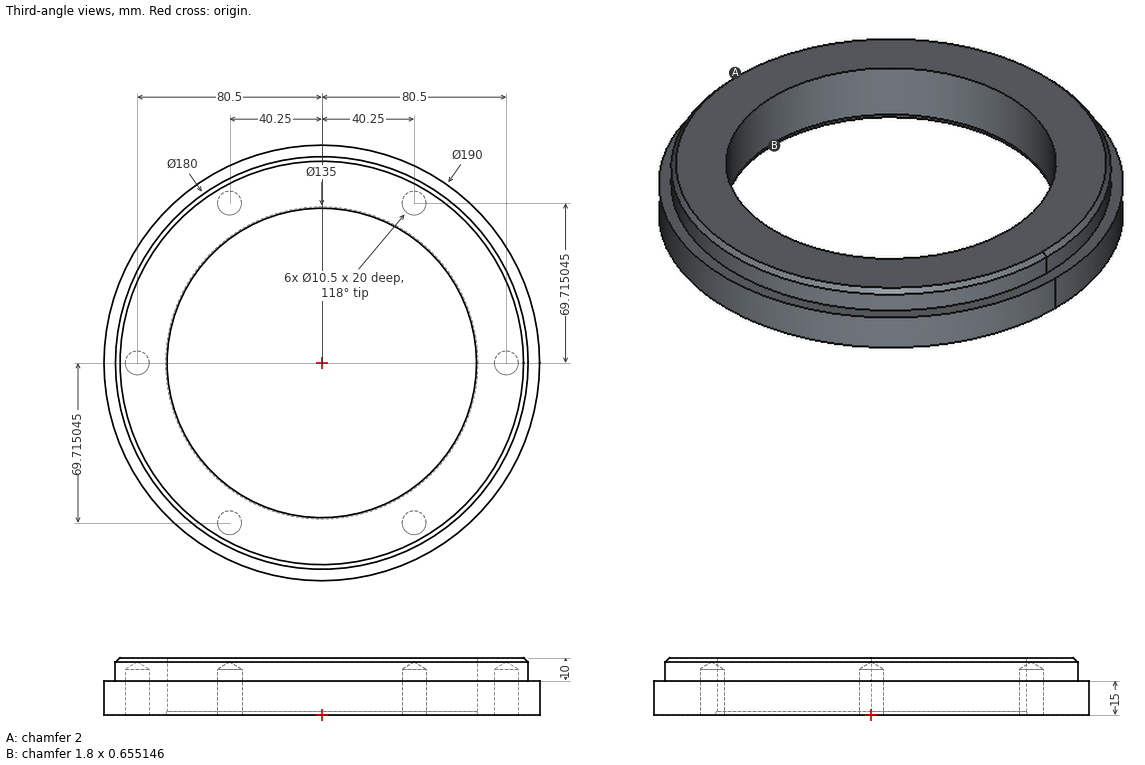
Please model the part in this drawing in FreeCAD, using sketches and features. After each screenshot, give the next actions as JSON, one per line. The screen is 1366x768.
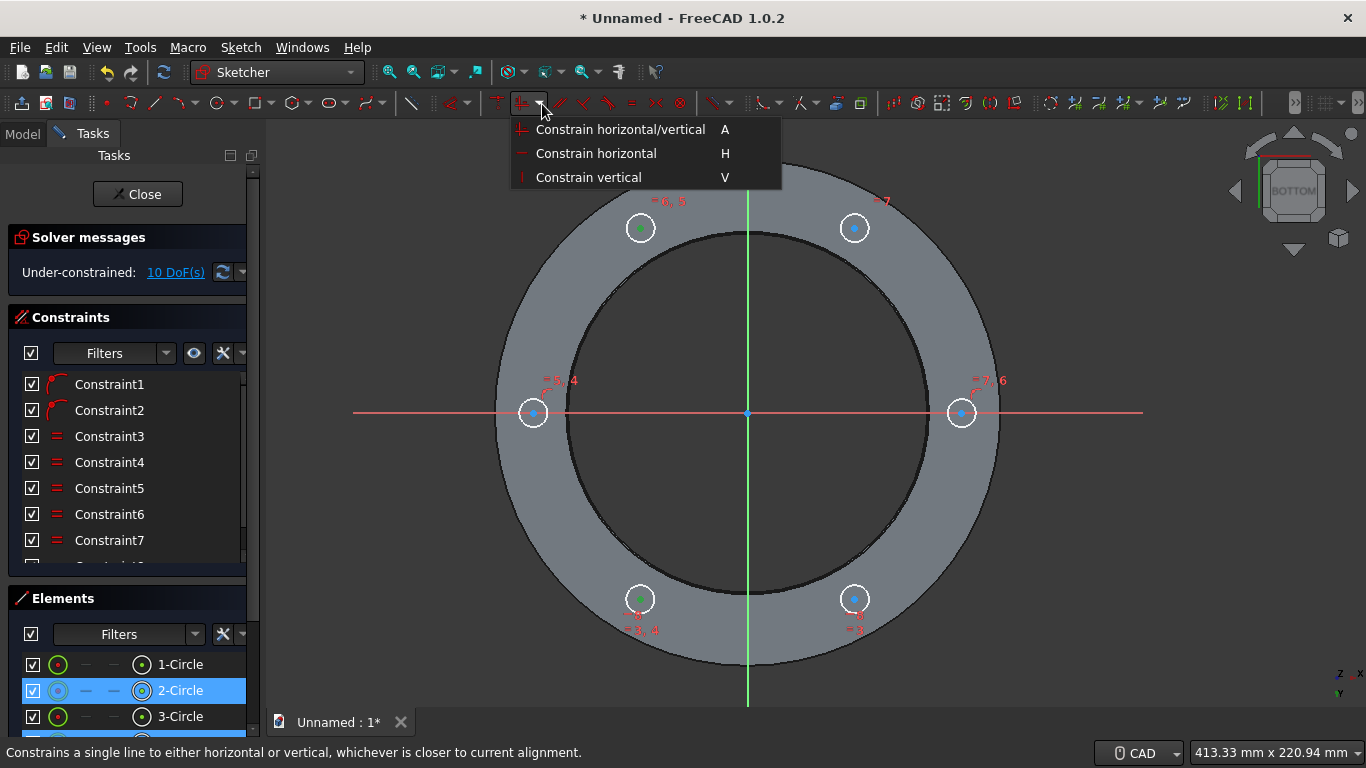
{"action": "left_click", "coordinate": [646, 177]}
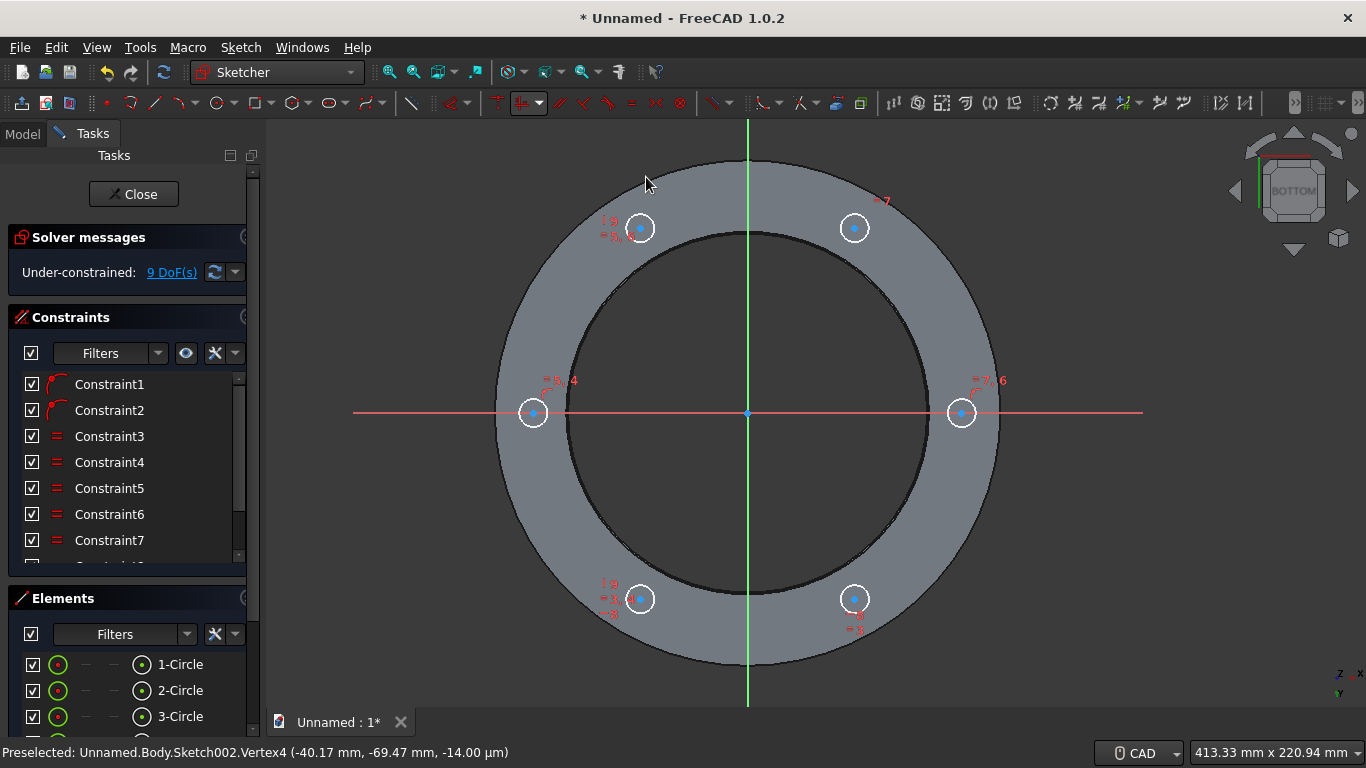
{"action": "left_click", "coordinate": [855, 599]}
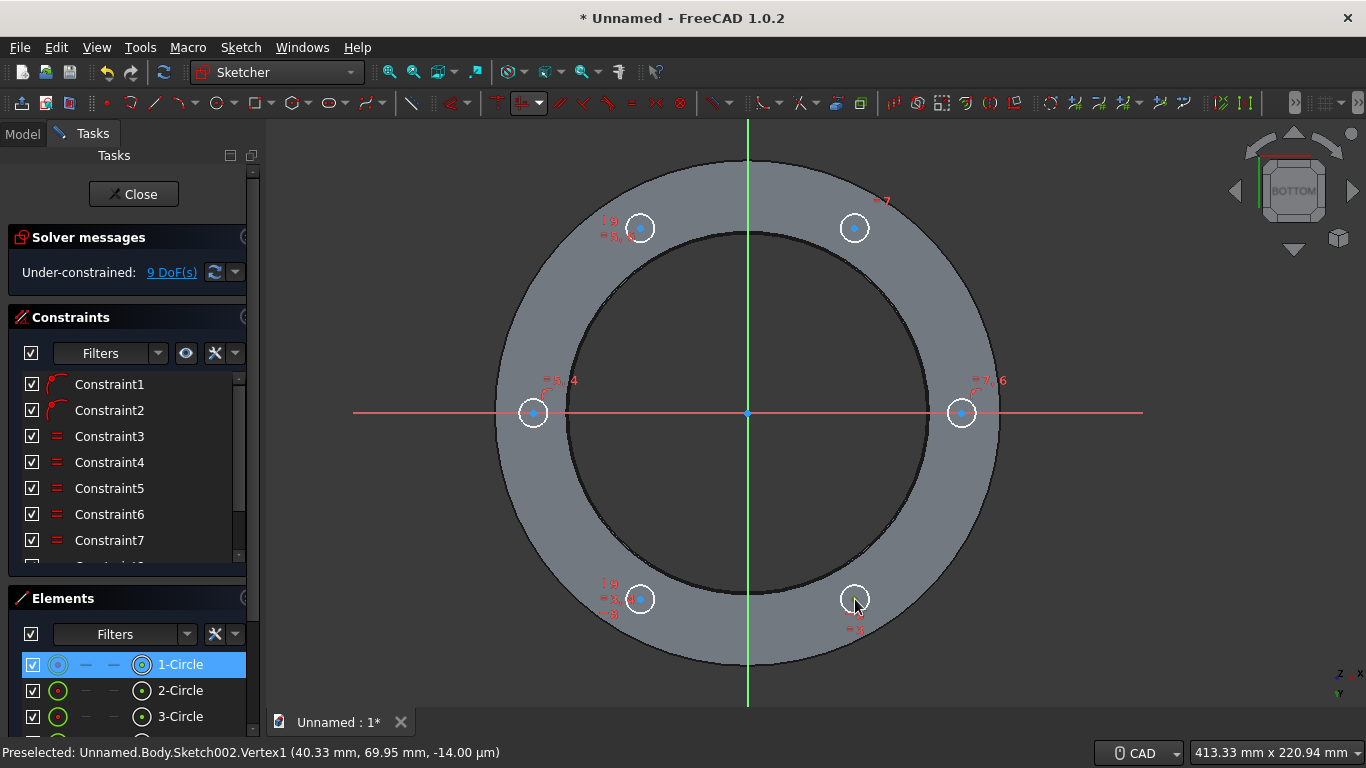
{"action": "left_click", "coordinate": [855, 228]}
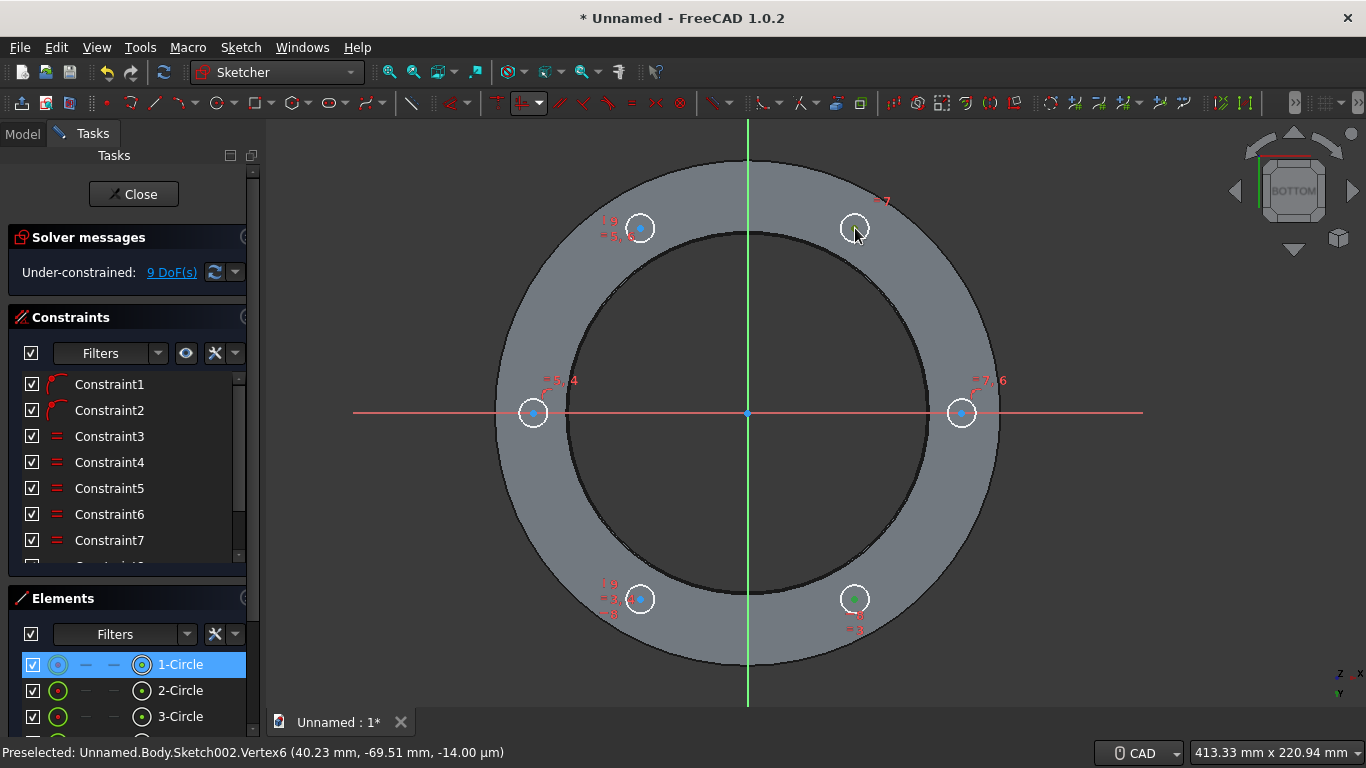
{"action": "key", "text": "v"}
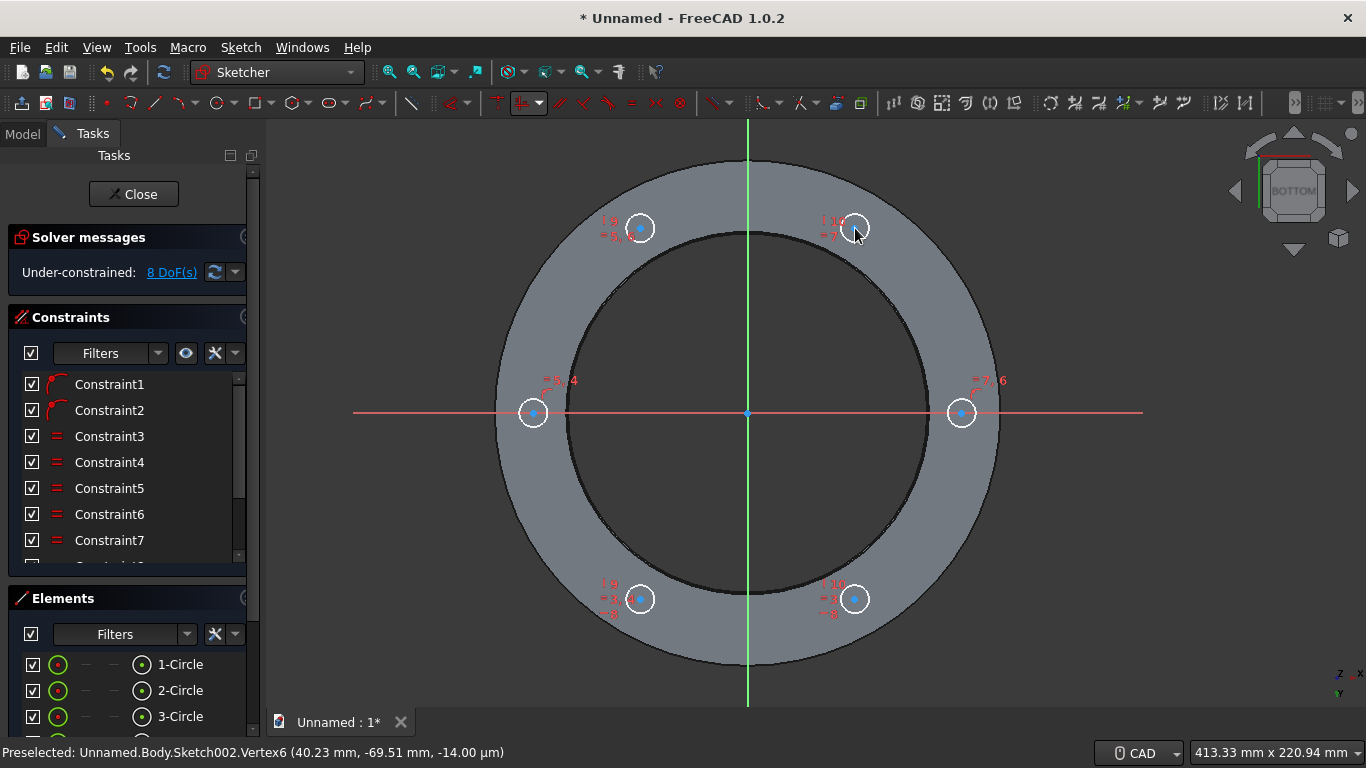
{"action": "left_click", "coordinate": [640, 228]}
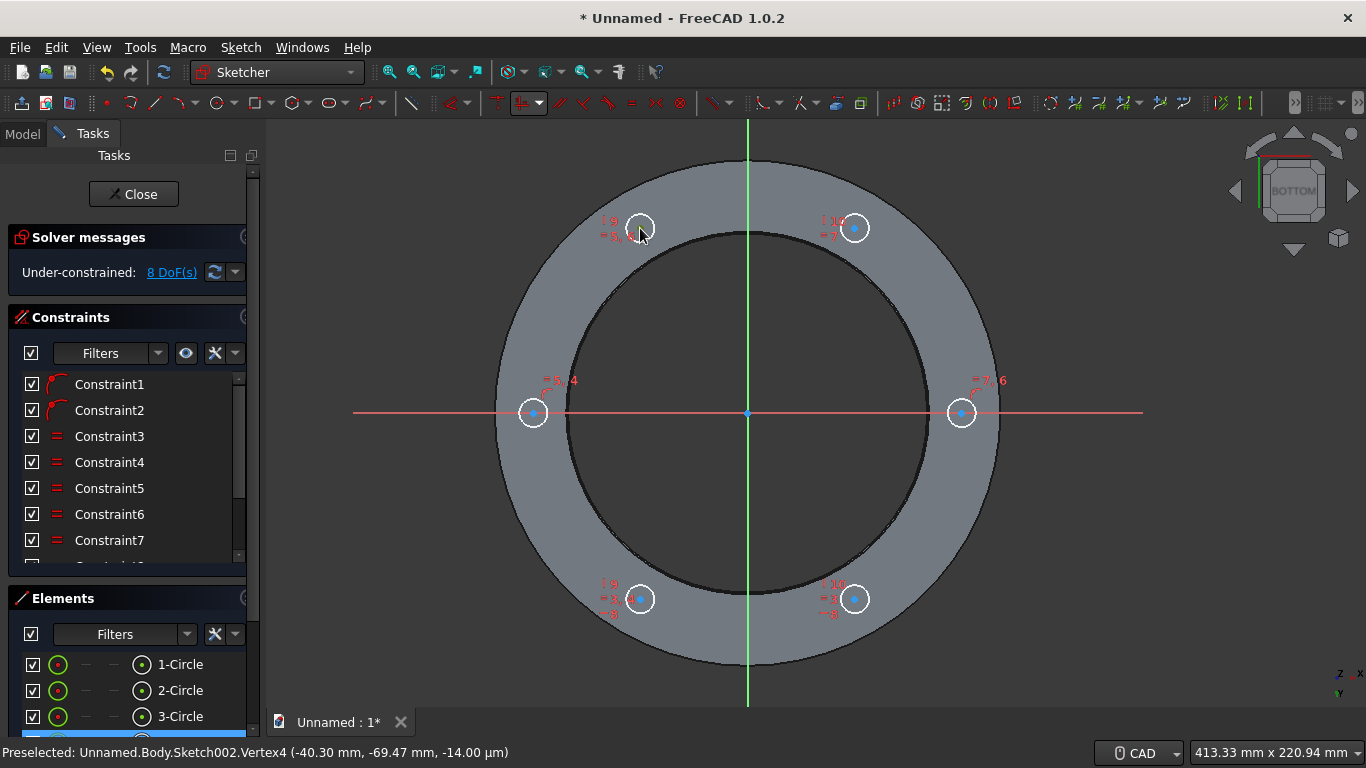
{"action": "left_click", "coordinate": [855, 228]}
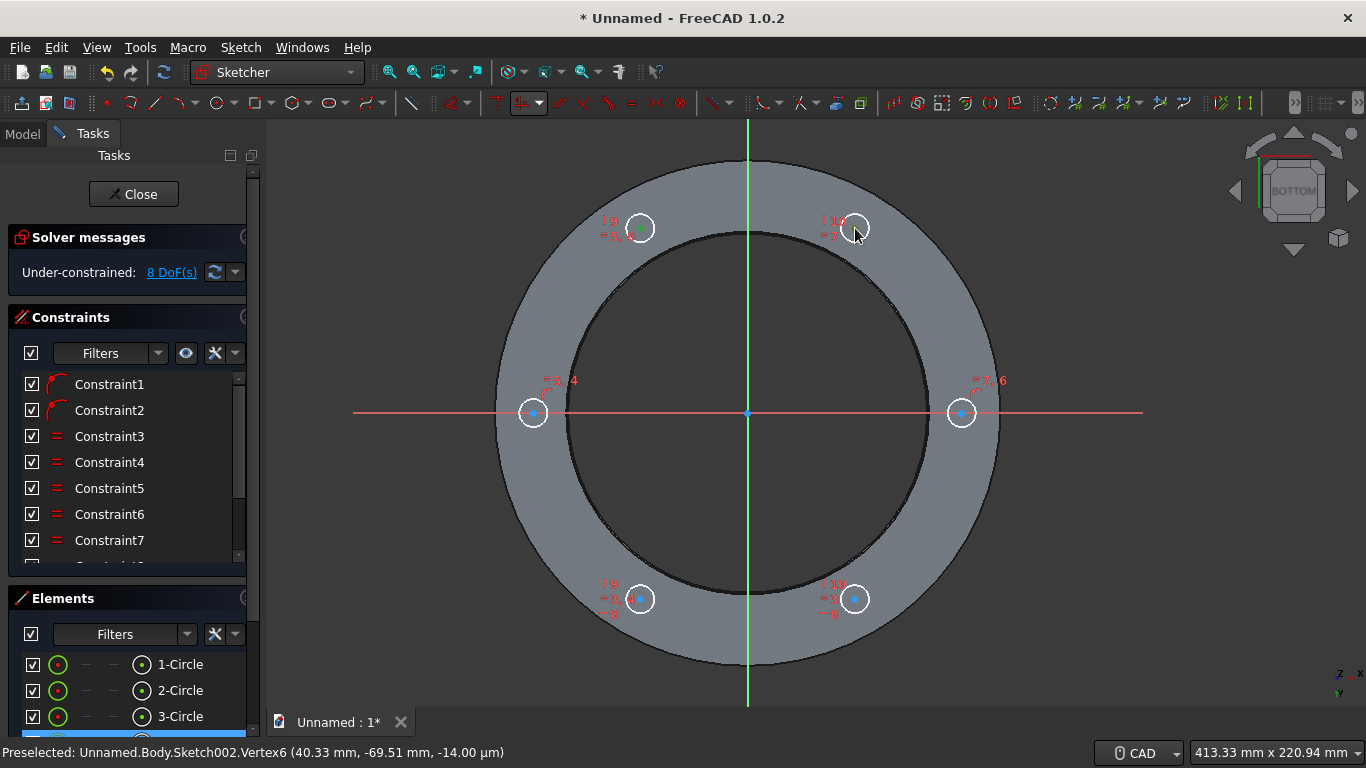
{"action": "key", "text": "h"}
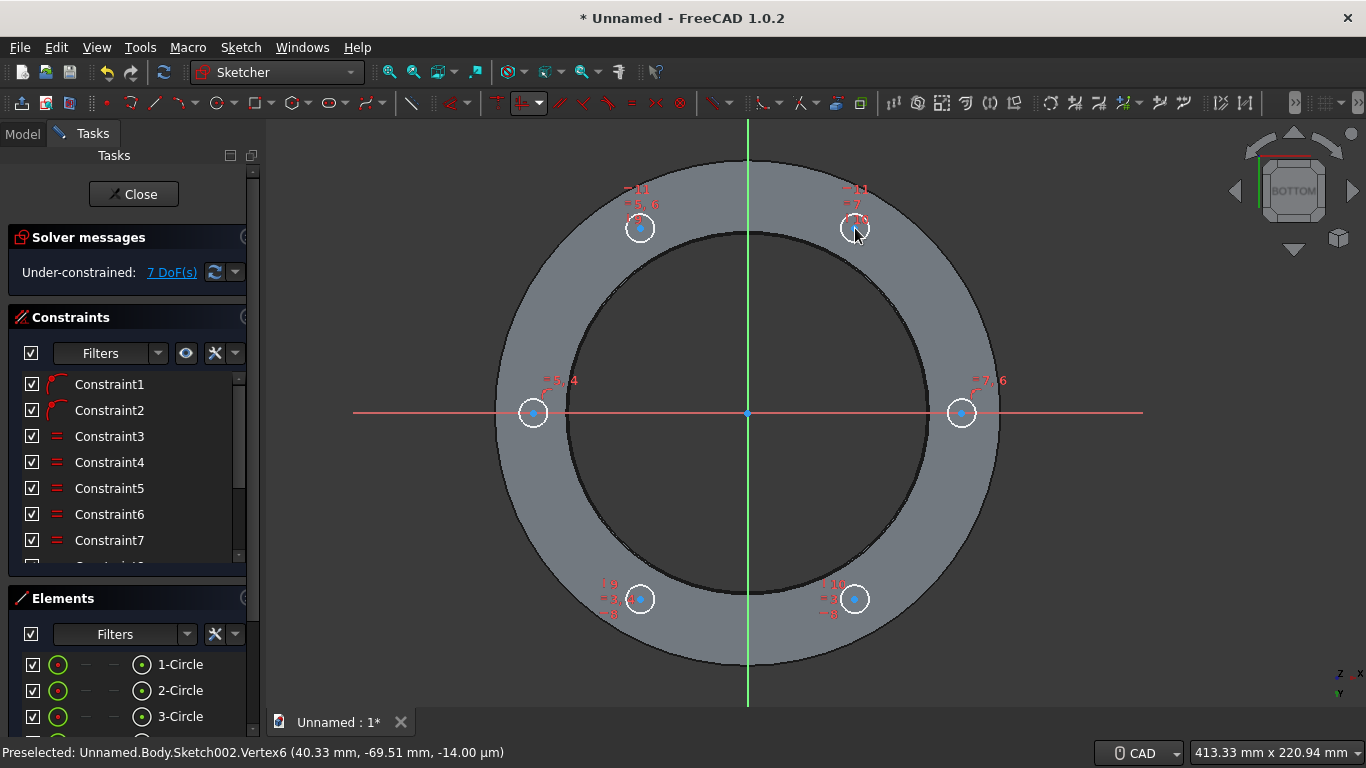
{"action": "left_click", "coordinate": [450, 104]}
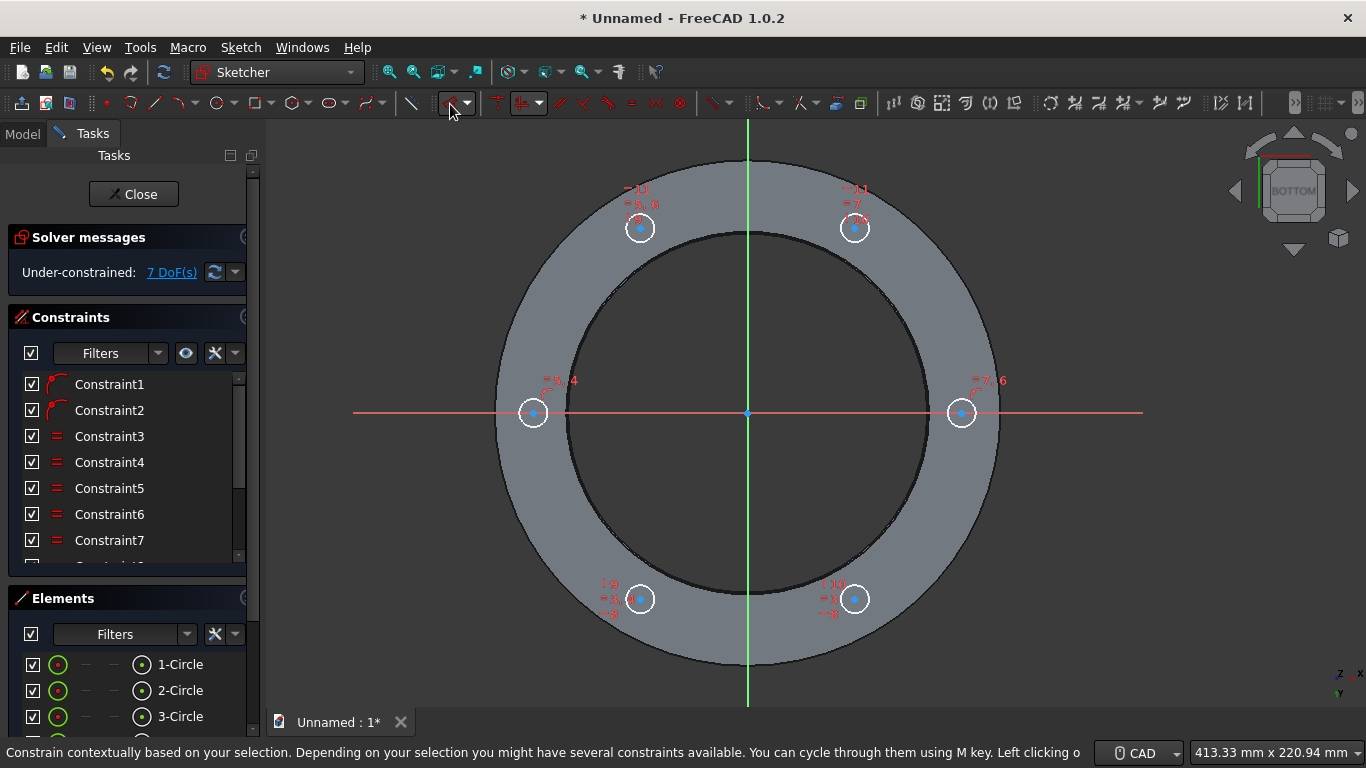
{"action": "scroll", "coordinate": [865, 589], "scroll_direction": "up", "scroll_amount": 2}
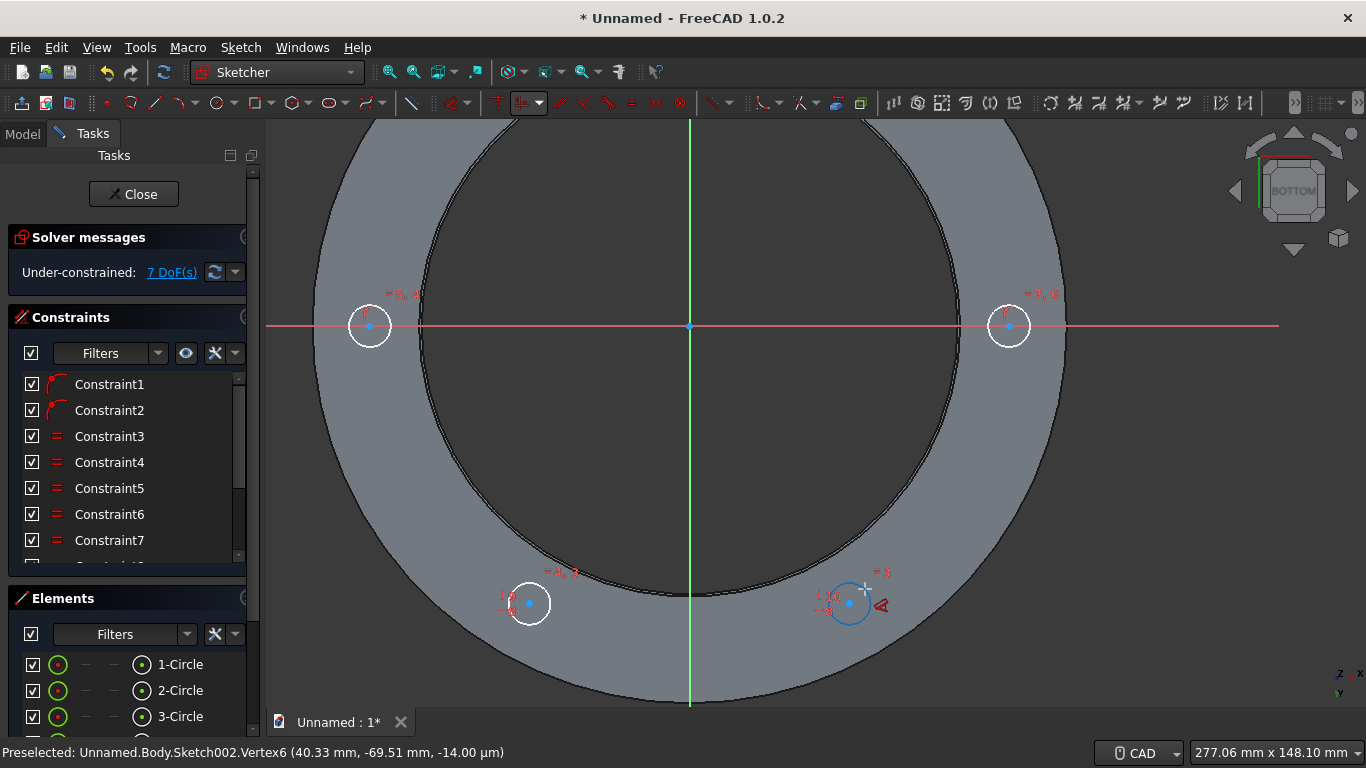
{"action": "left_click", "coordinate": [864, 589]}
{"action": "left_click", "coordinate": [886, 566]}